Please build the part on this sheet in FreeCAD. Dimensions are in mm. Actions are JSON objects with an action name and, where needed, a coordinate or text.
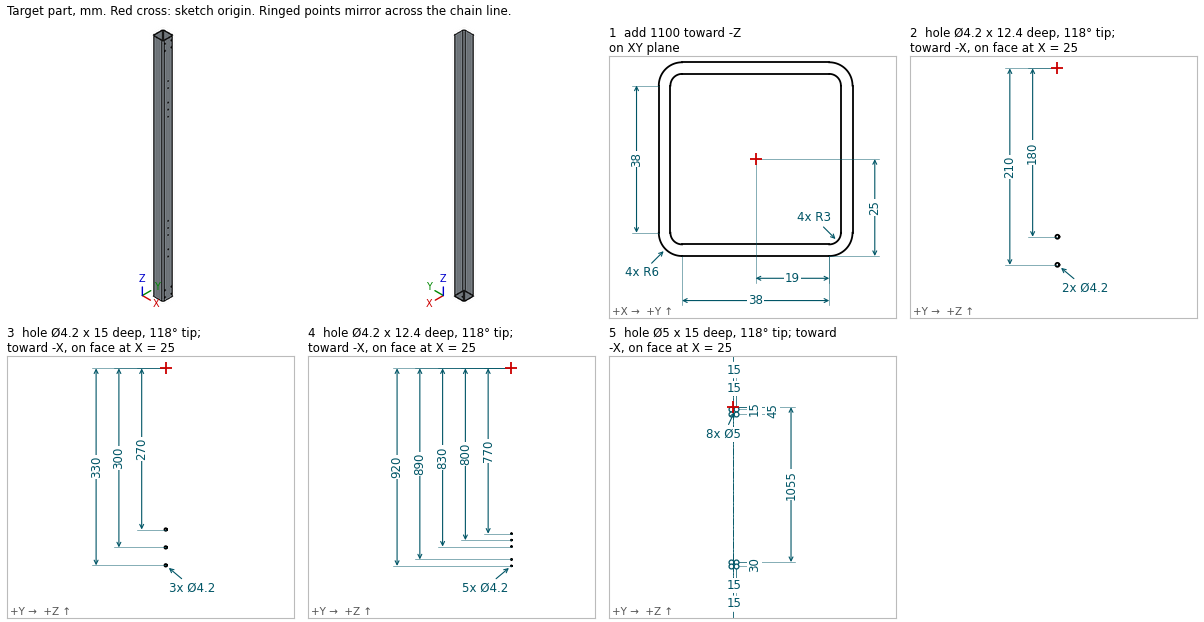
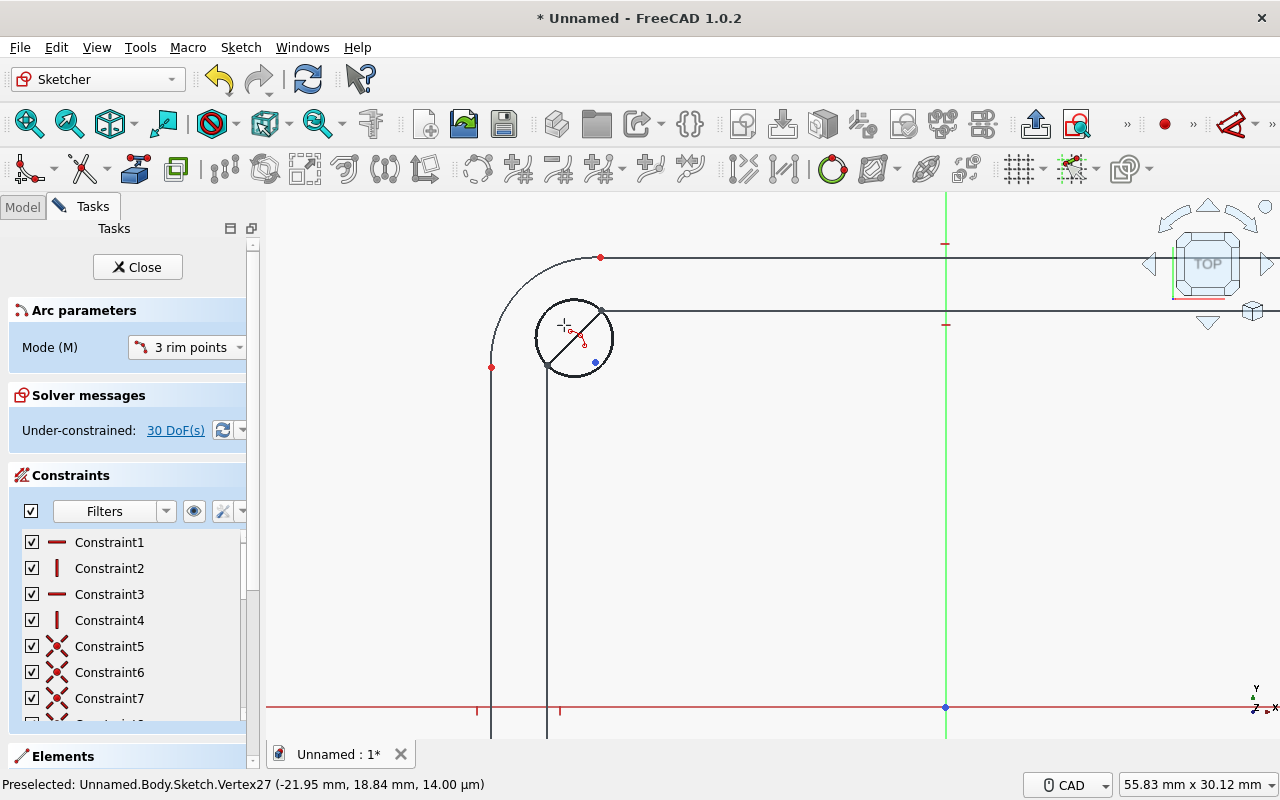
{"action": "left_click", "coordinate": [562, 324]}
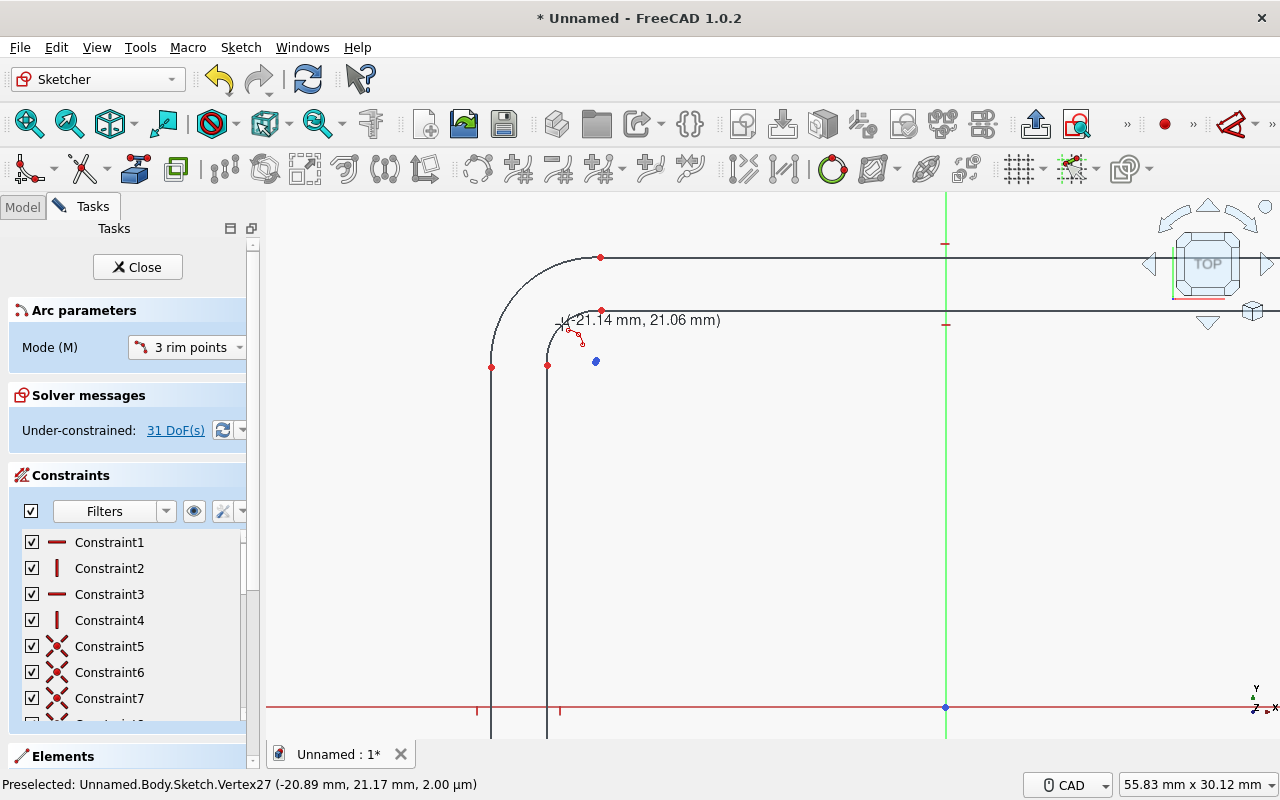
{"action": "scroll", "coordinate": [564, 325], "scroll_direction": "down", "scroll_amount": 5}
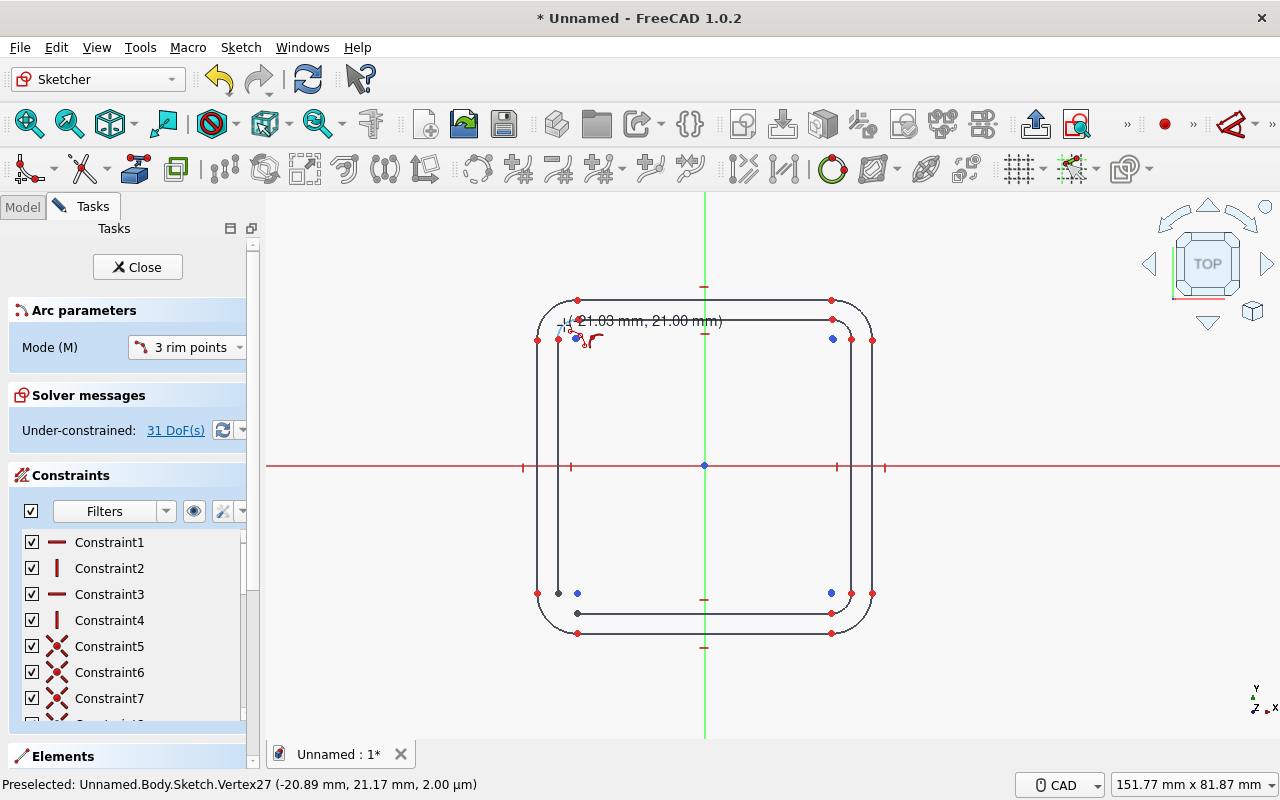
{"action": "left_click", "coordinate": [558, 594]}
{"action": "left_click", "coordinate": [578, 614]}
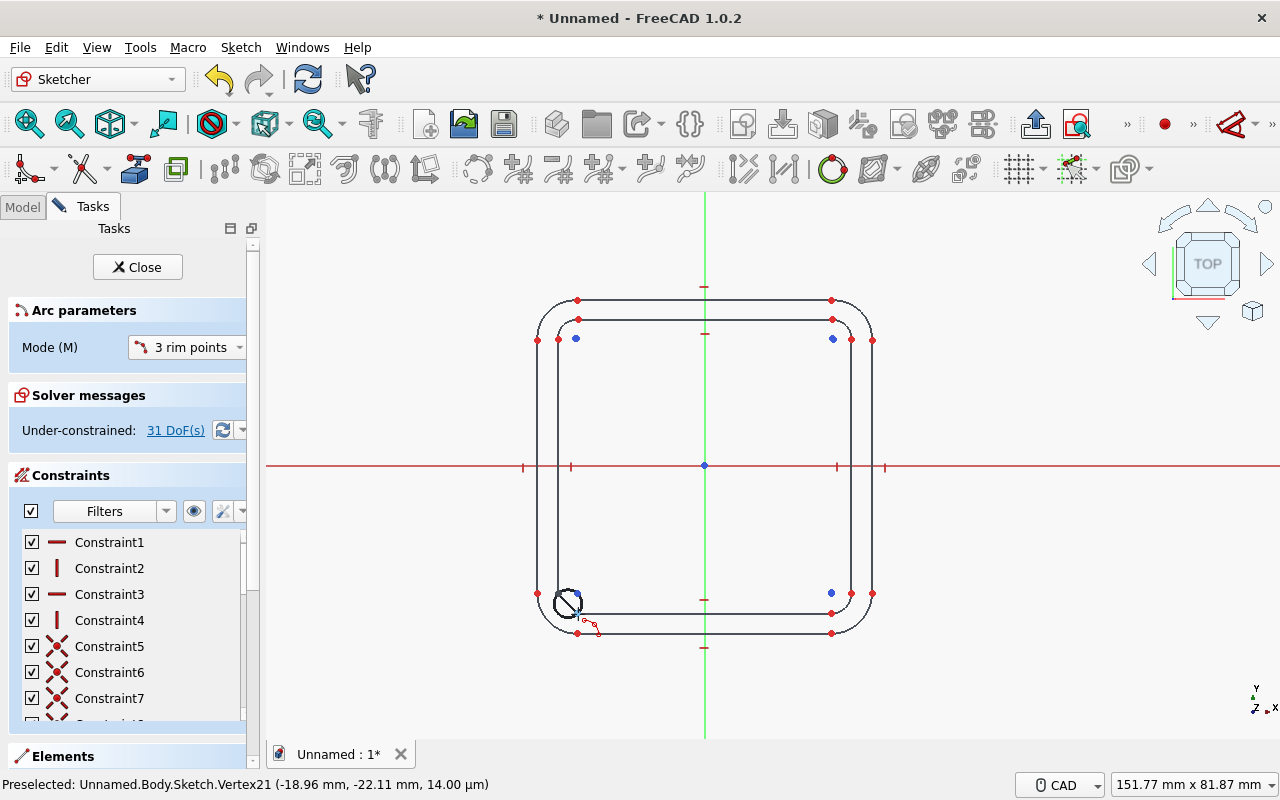
{"action": "scroll", "coordinate": [564, 607], "scroll_direction": "up", "scroll_amount": 5}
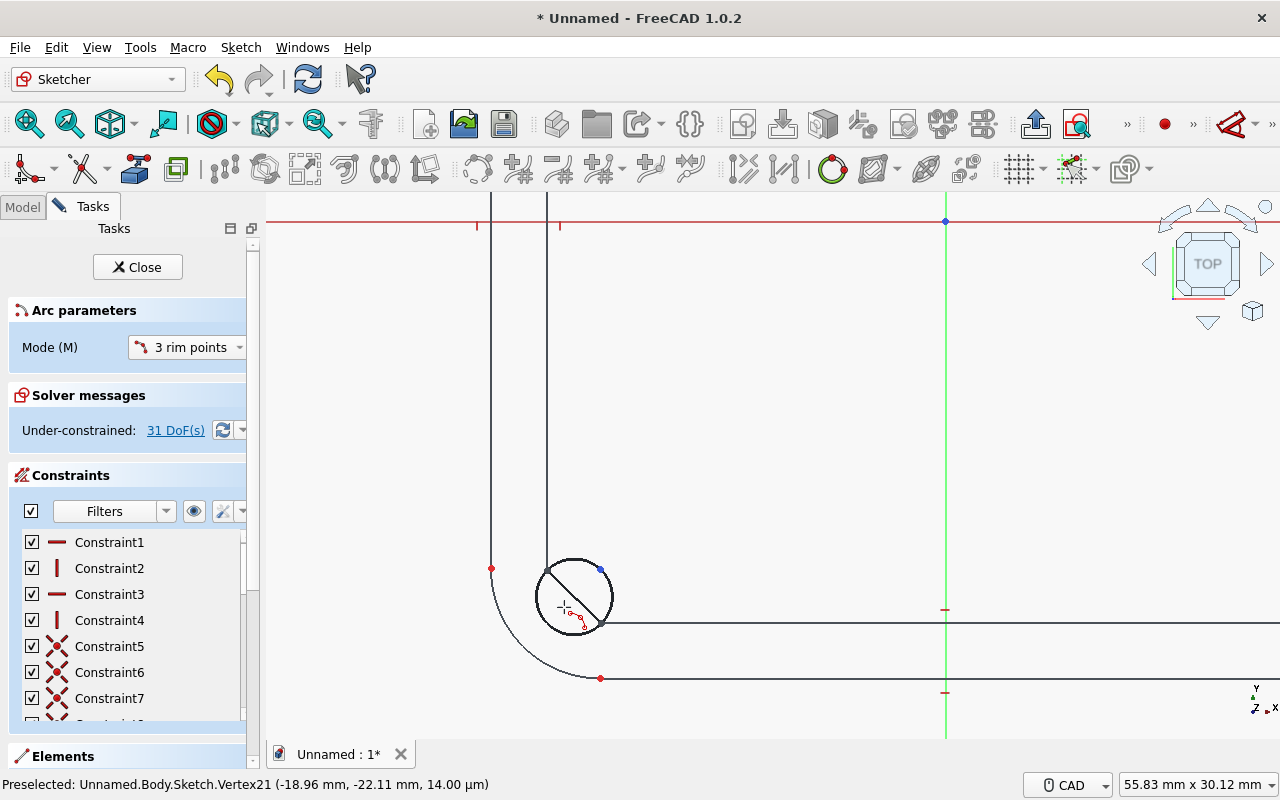
{"action": "left_click", "coordinate": [562, 606]}
{"action": "key", "text": "Escape"}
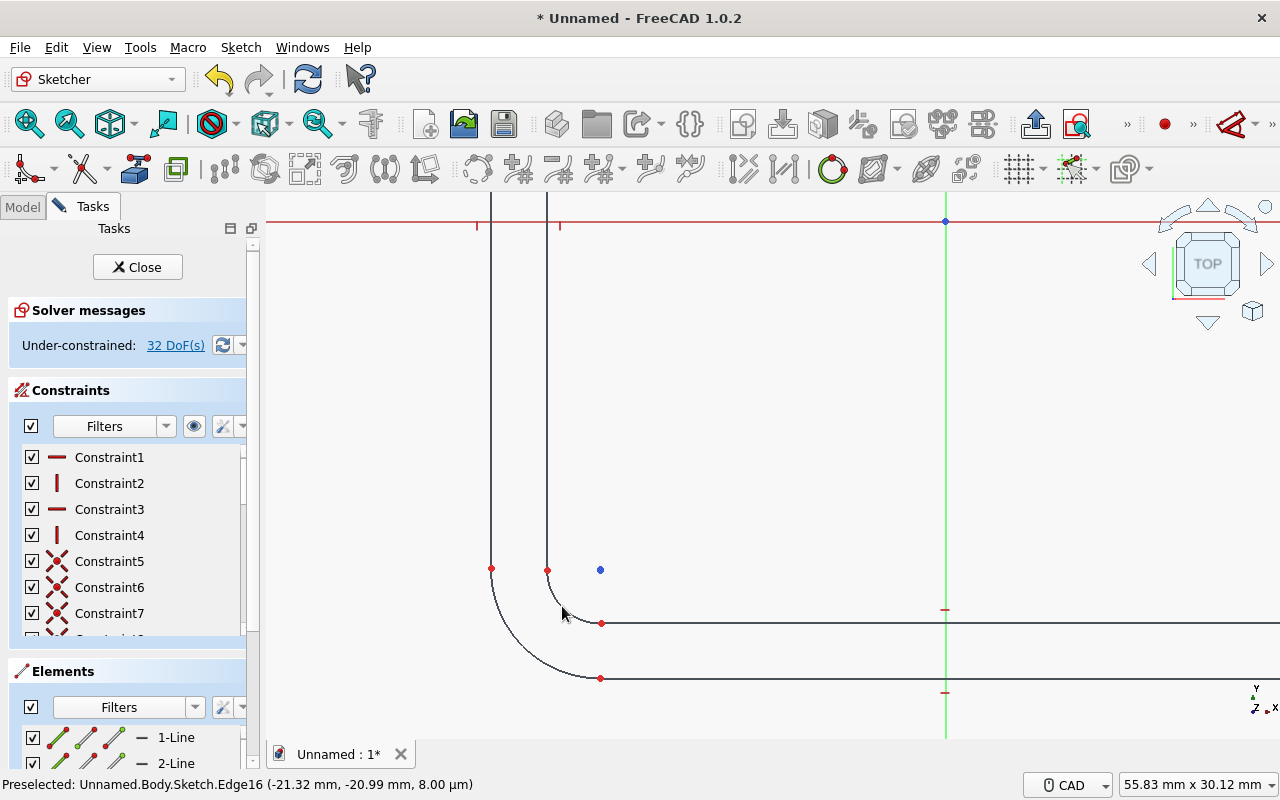
{"action": "left_click", "coordinate": [1084, 679]}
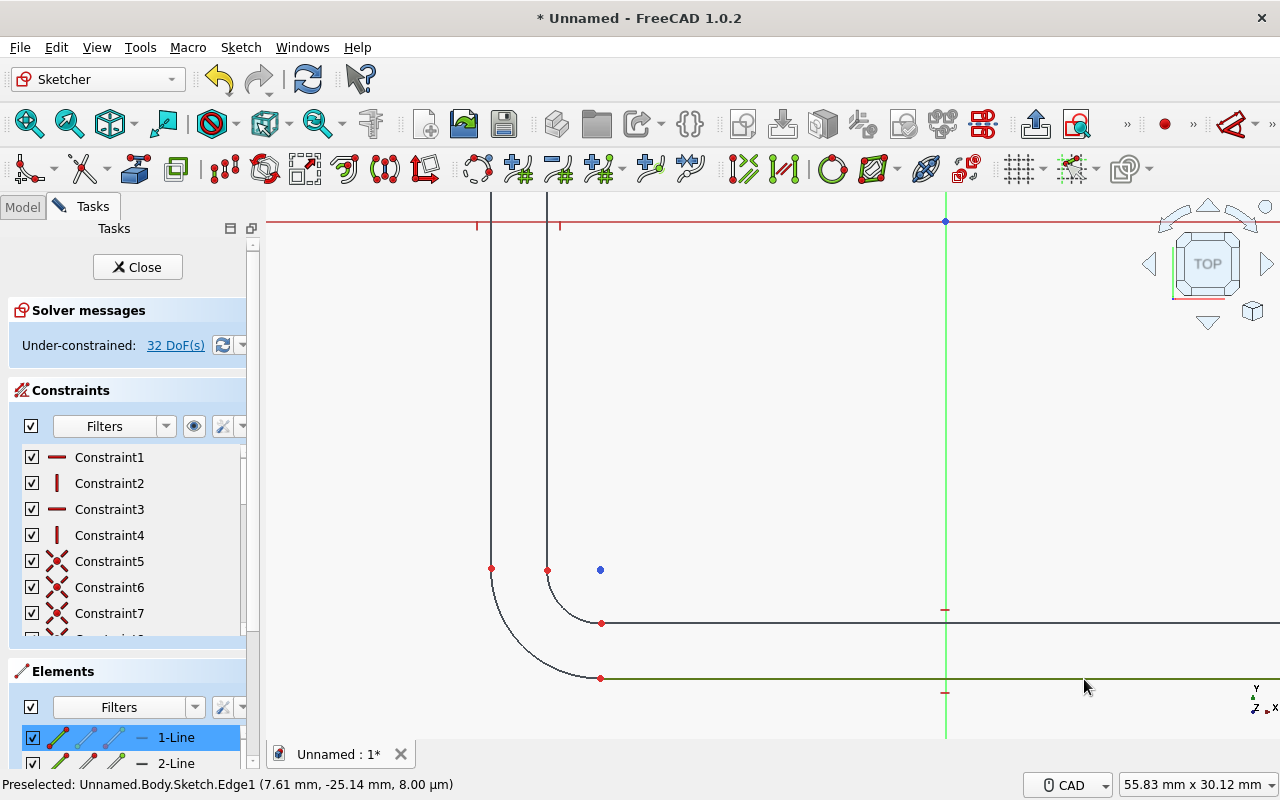
{"action": "left_click", "coordinate": [503, 619]}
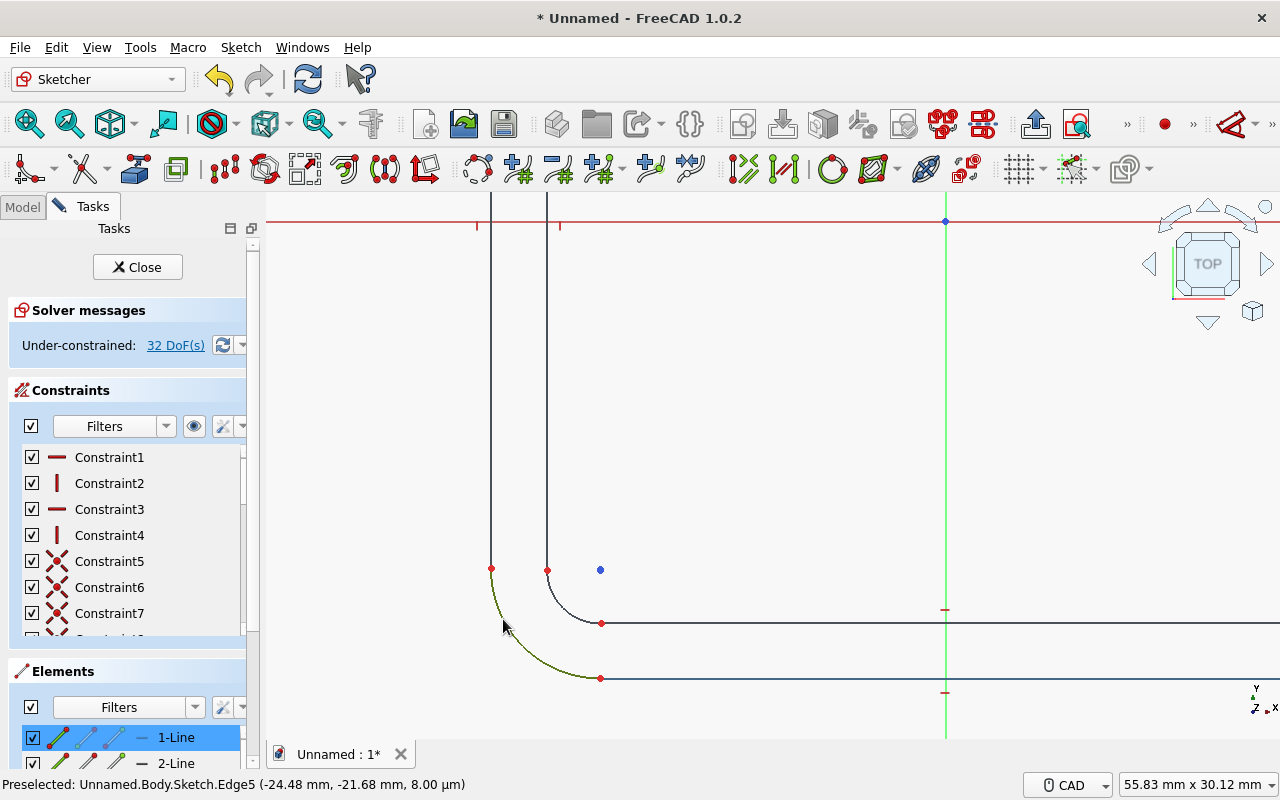
{"action": "key", "text": "t"}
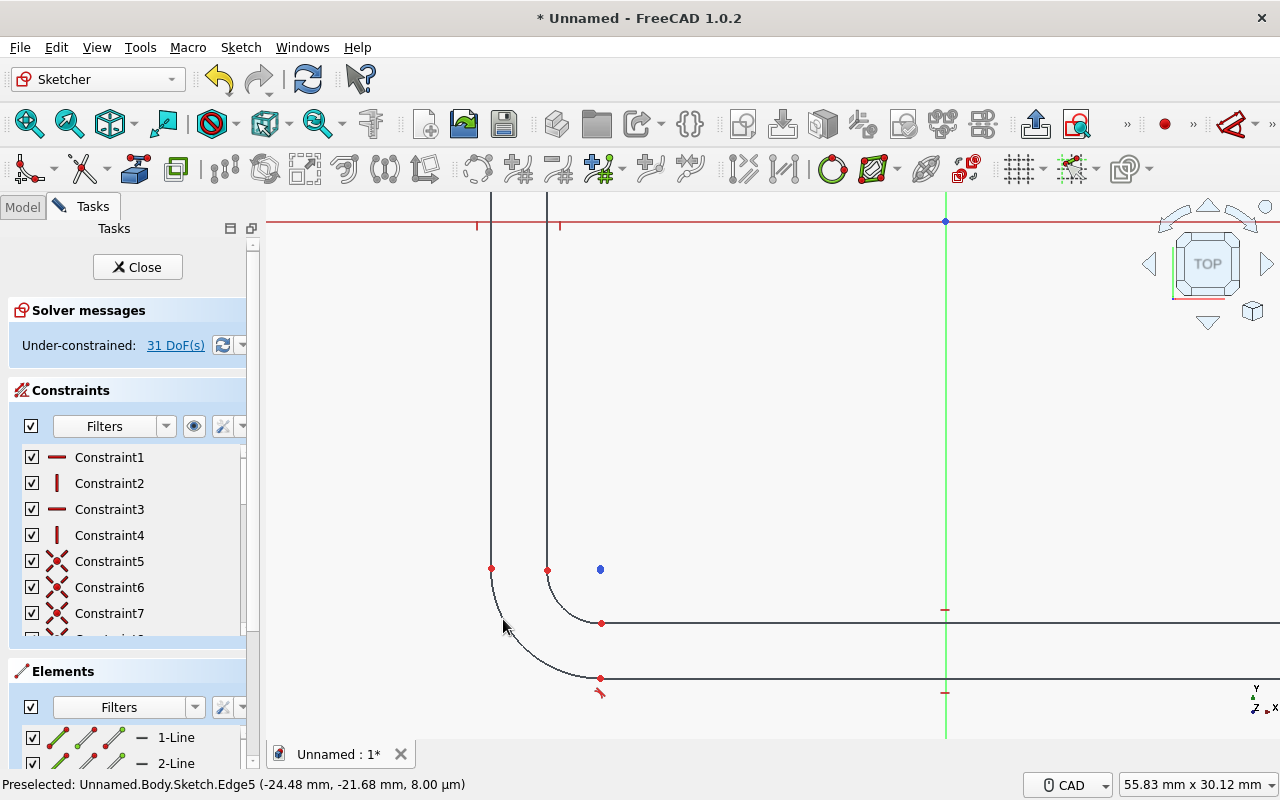
{"action": "left_click", "coordinate": [1084, 679]}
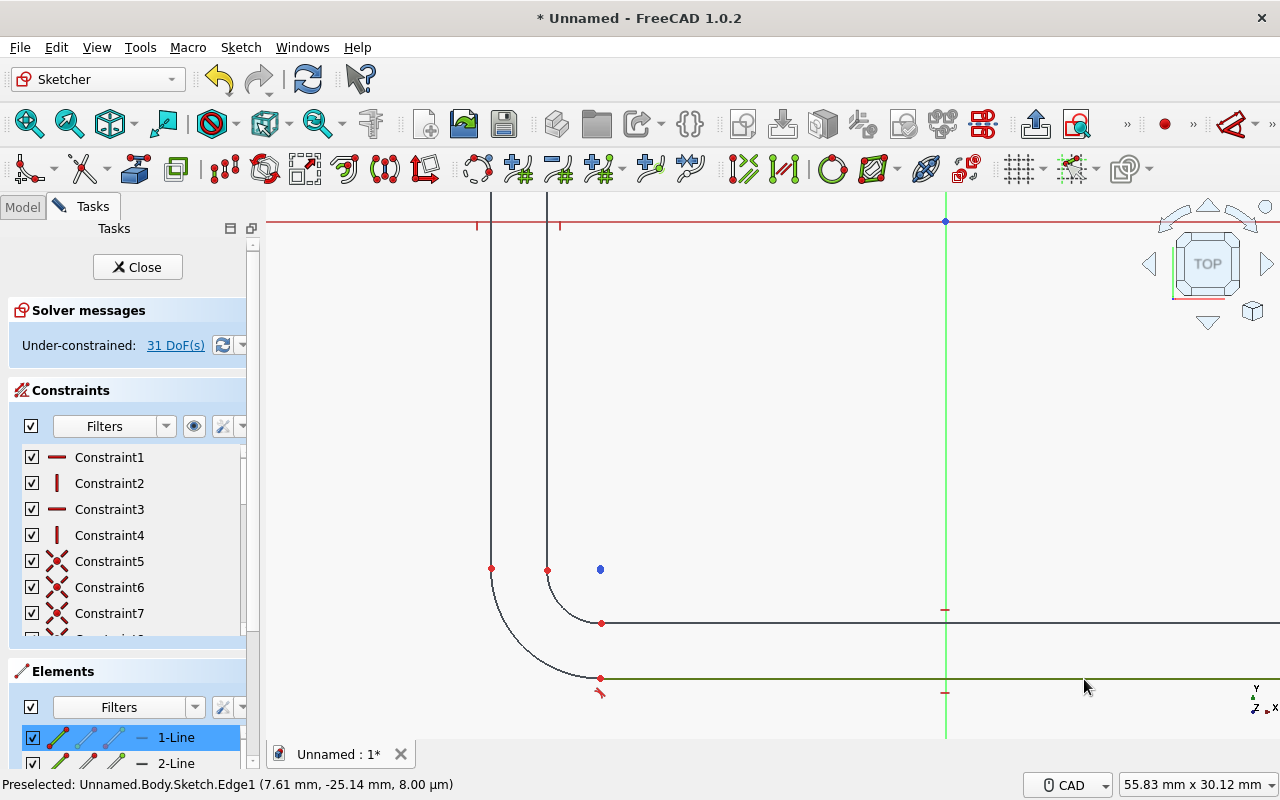
{"action": "scroll", "coordinate": [564, 607], "scroll_direction": "down", "scroll_amount": 5}